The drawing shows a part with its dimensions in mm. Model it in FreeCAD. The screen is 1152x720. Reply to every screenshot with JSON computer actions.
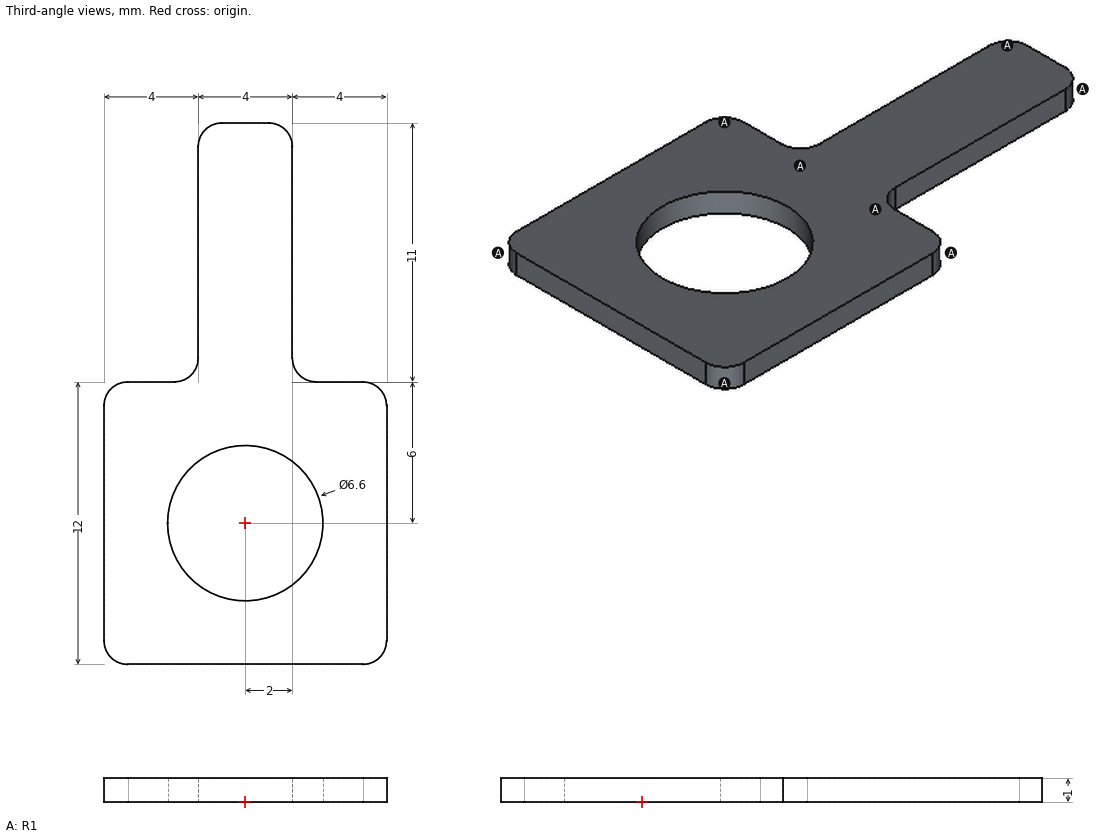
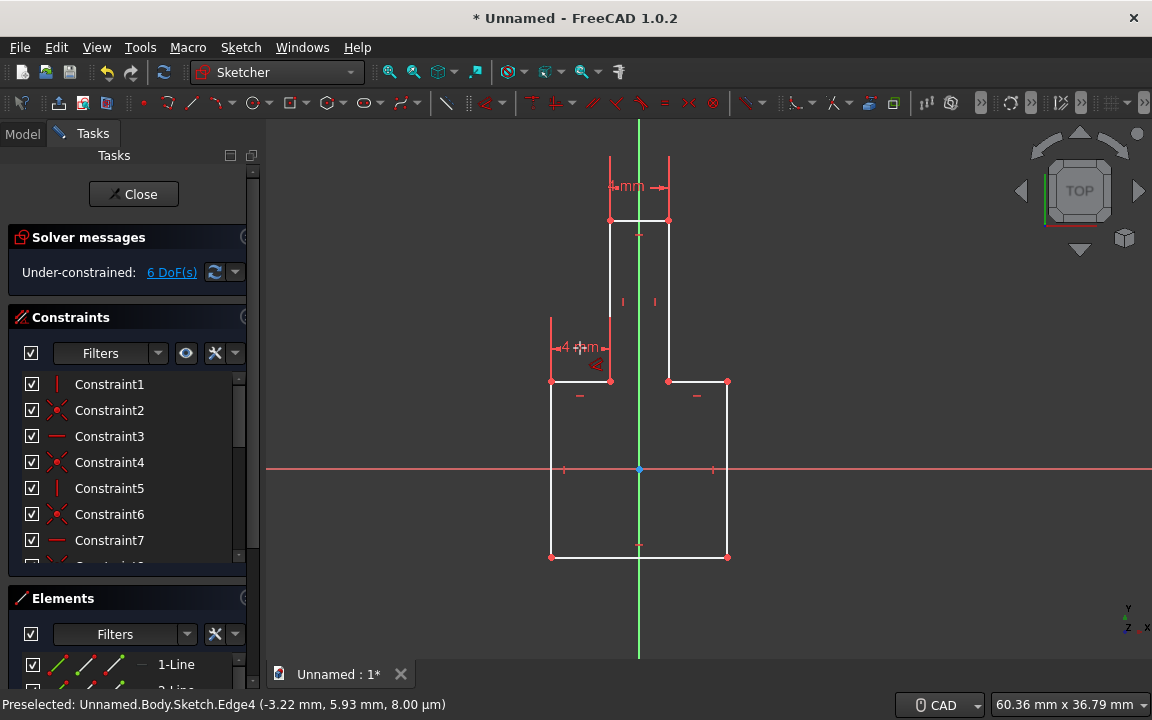
{"action": "left_click", "coordinate": [710, 382]}
{"action": "left_click", "coordinate": [698, 348]}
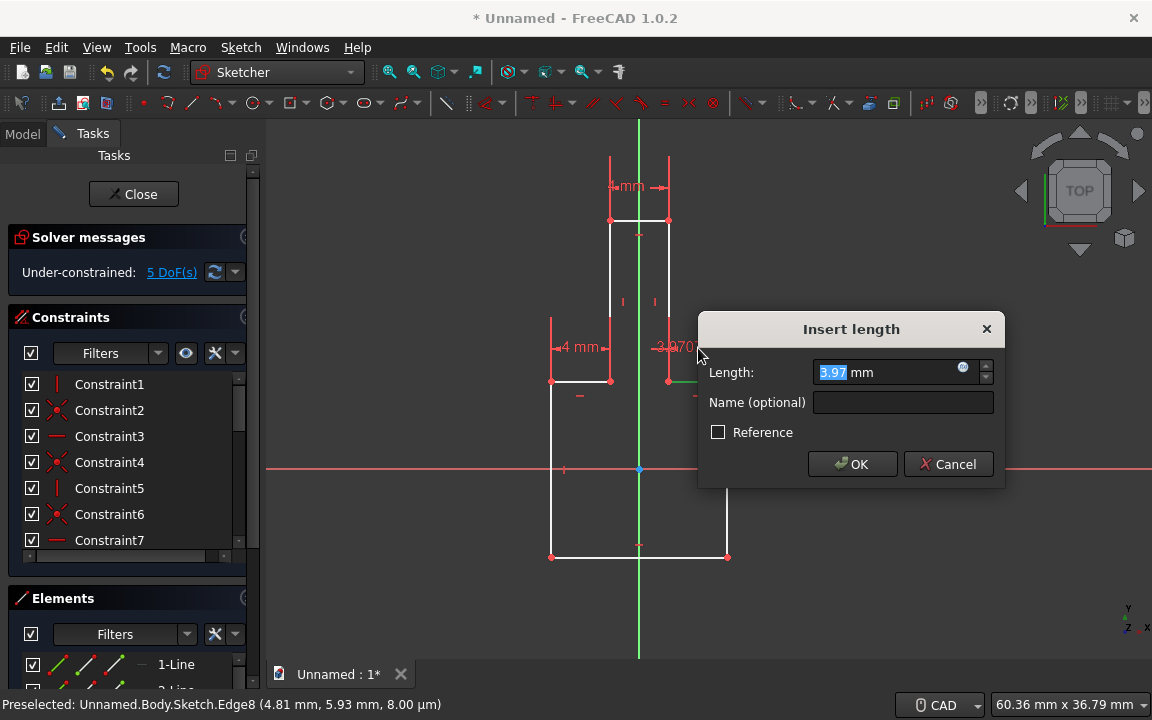
{"action": "type", "text": "4"}
{"action": "key", "text": "Return"}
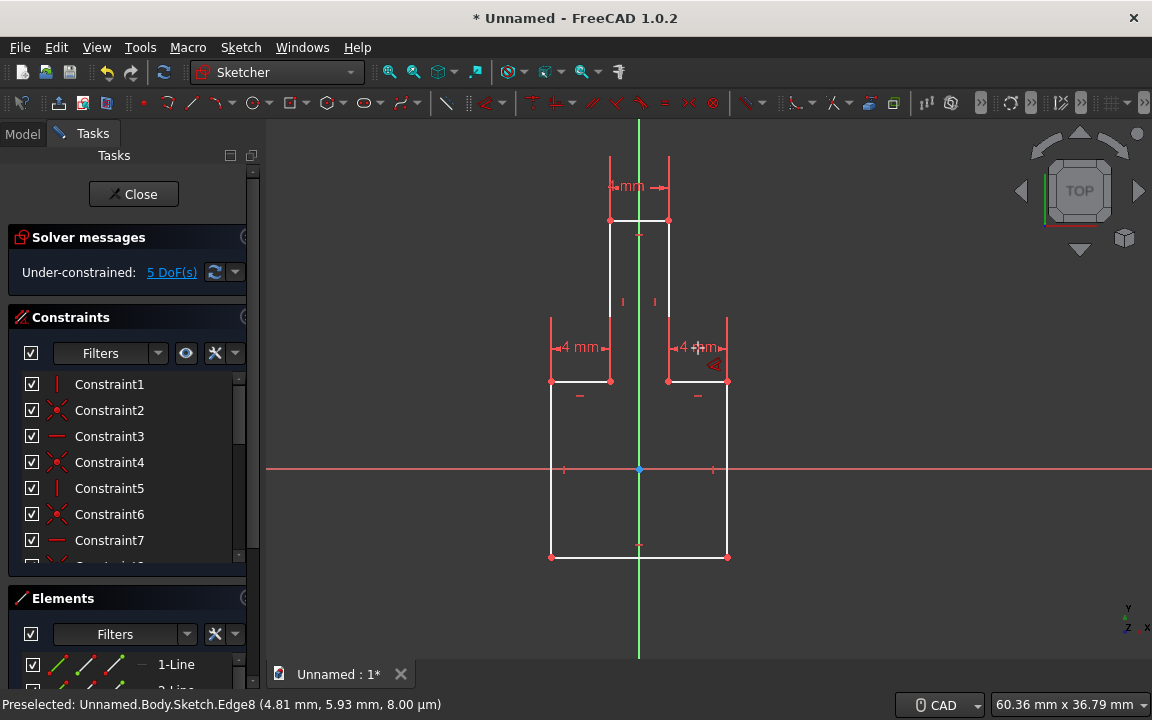
{"action": "left_click", "coordinate": [669, 334]}
{"action": "left_click", "coordinate": [703, 302]}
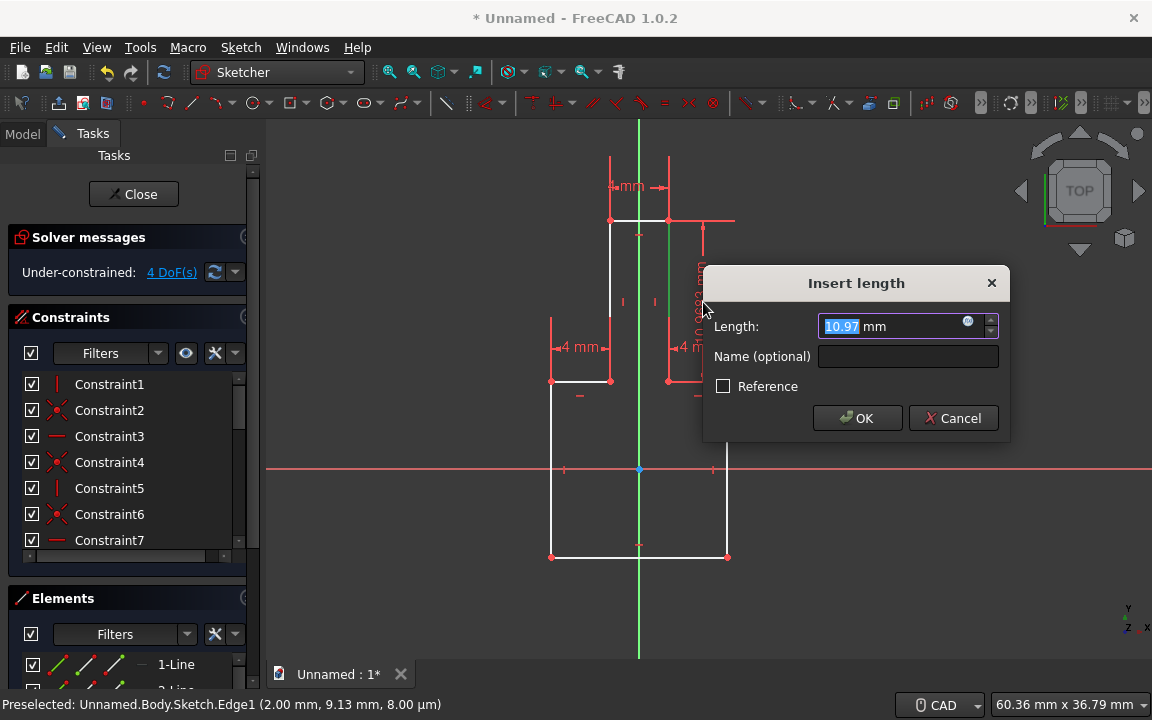
{"action": "type", "text": "11"}
{"action": "key", "text": "Return"}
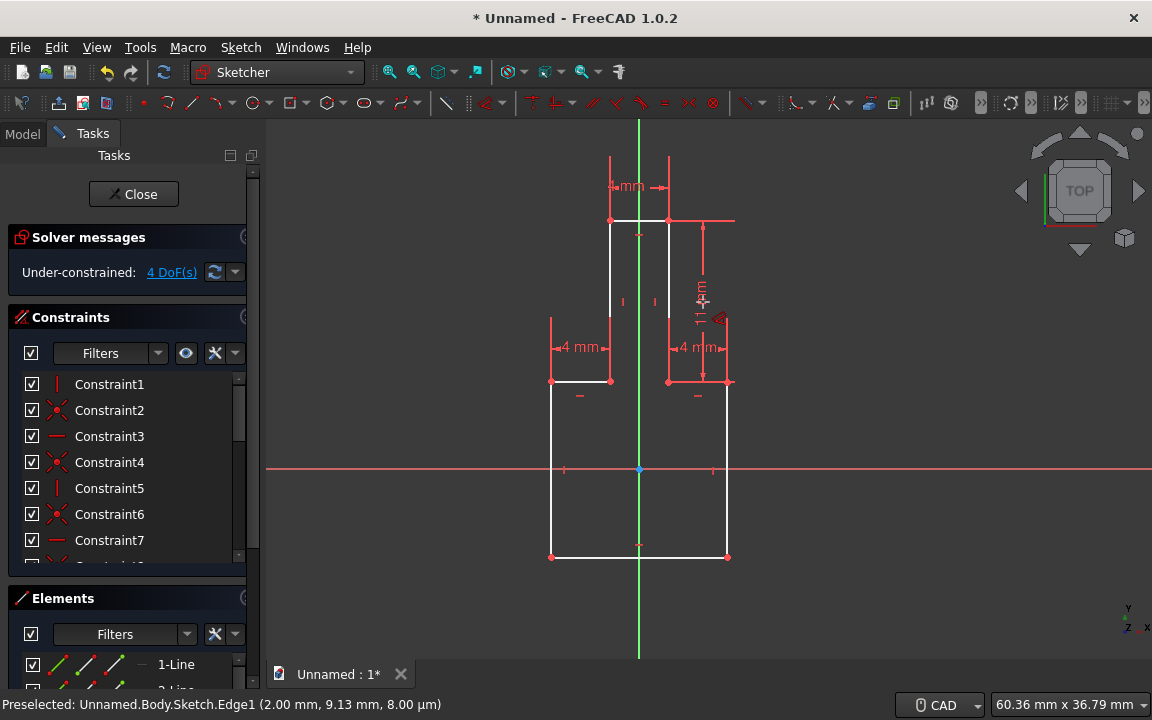
{"action": "left_click", "coordinate": [610, 269]}
{"action": "left_click", "coordinate": [576, 302]}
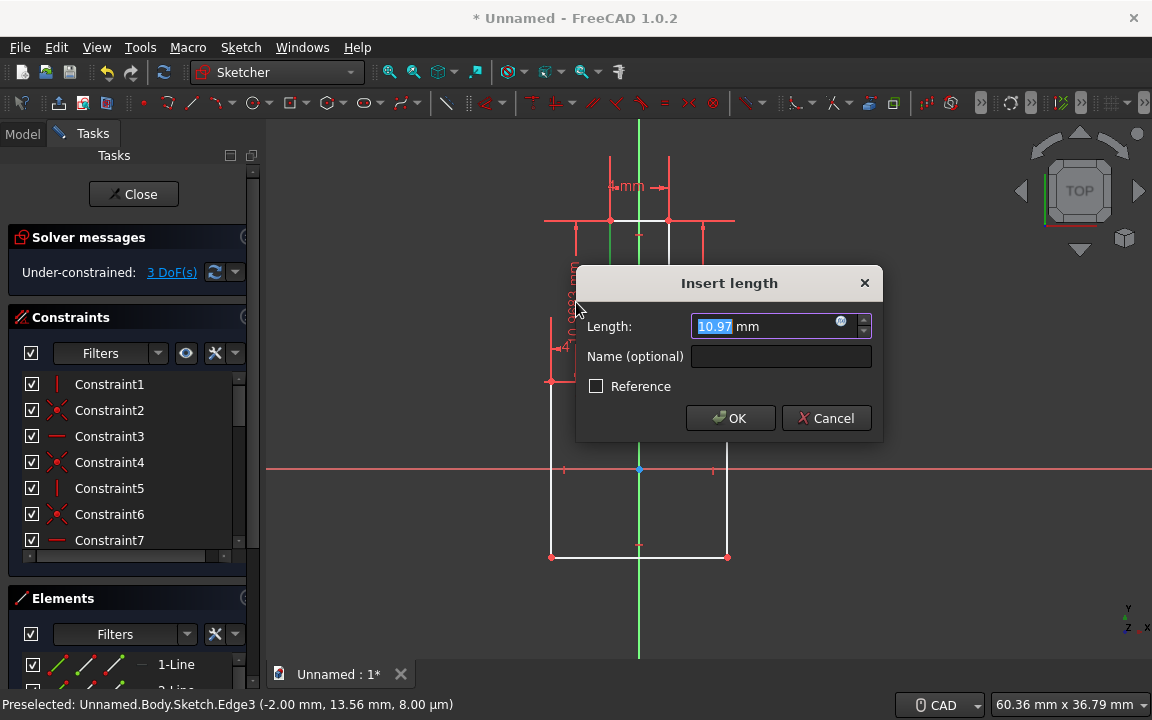
{"action": "type", "text": "11"}
{"action": "key", "text": "Return"}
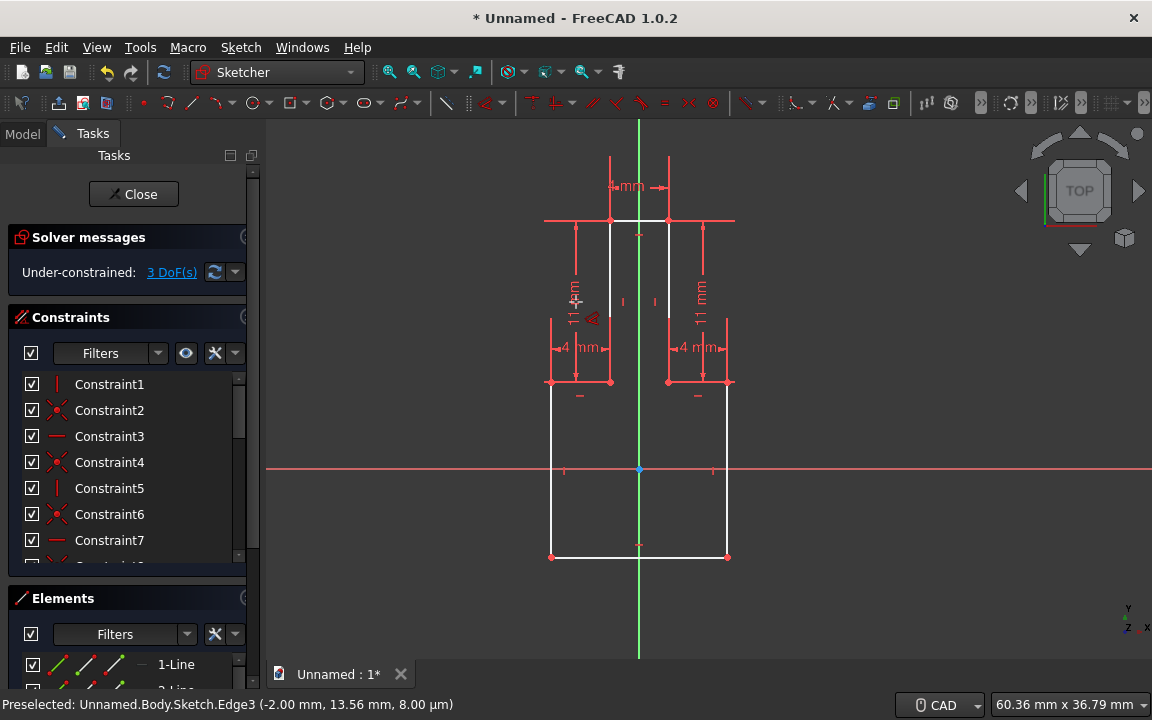
{"action": "left_click", "coordinate": [551, 435]}
{"action": "left_click", "coordinate": [517, 430]}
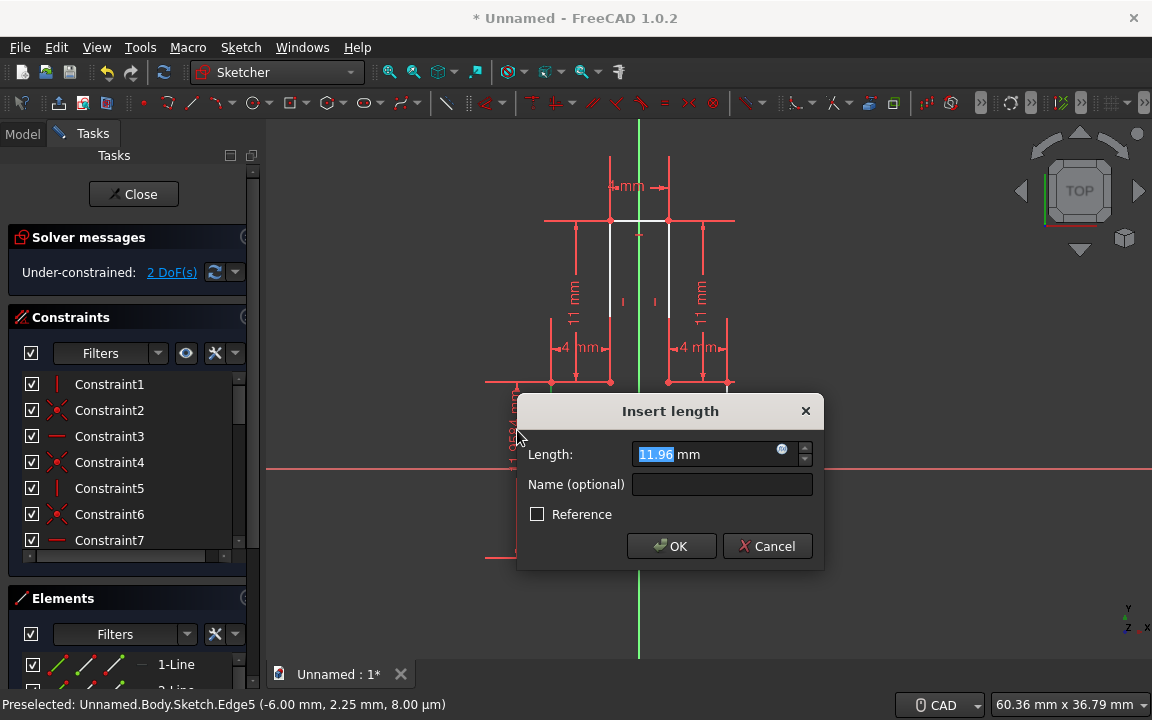
{"action": "type", "text": "12"}
{"action": "key", "text": "Return"}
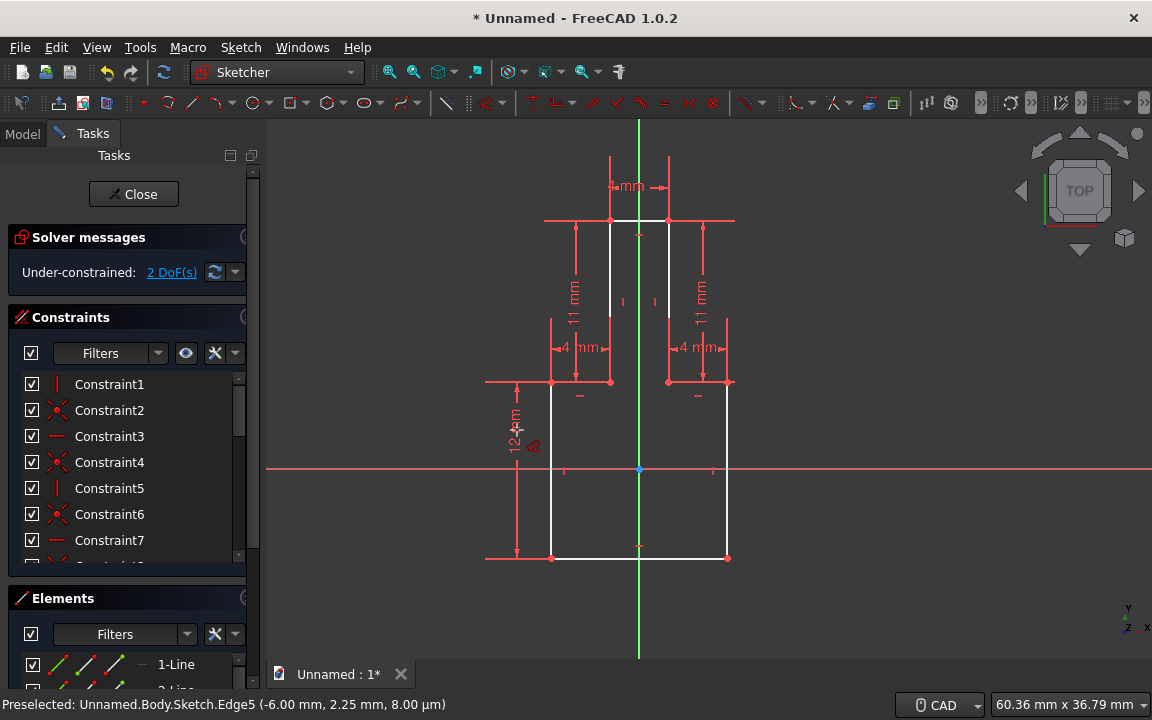
{"action": "scroll", "coordinate": [669, 382], "scroll_direction": "up", "scroll_amount": 2}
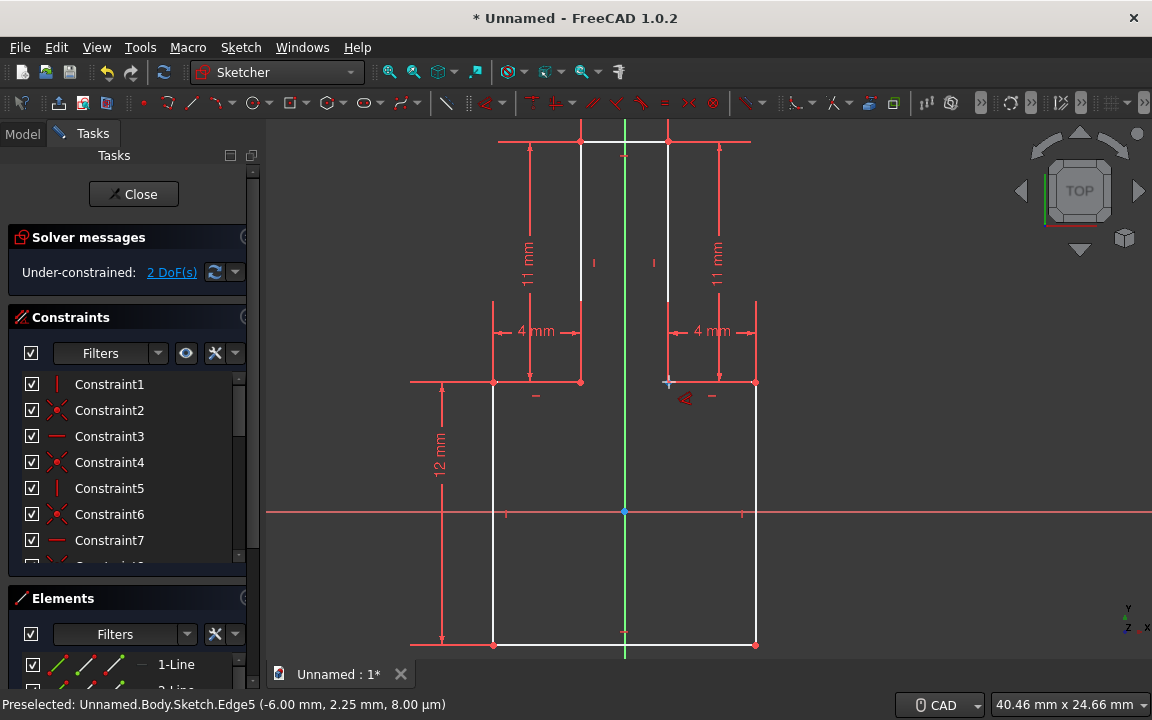
{"action": "left_click", "coordinate": [668, 382]}
{"action": "left_click", "coordinate": [646, 546]}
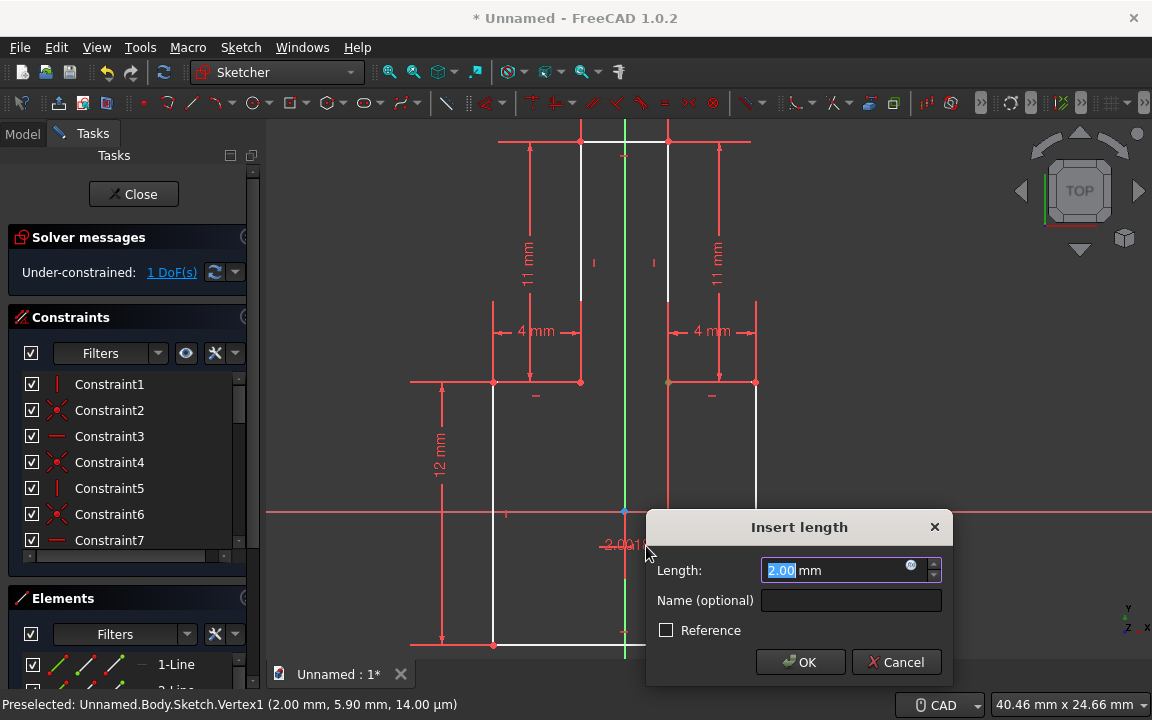
{"action": "type", "text": "2"}
{"action": "key", "text": "Return"}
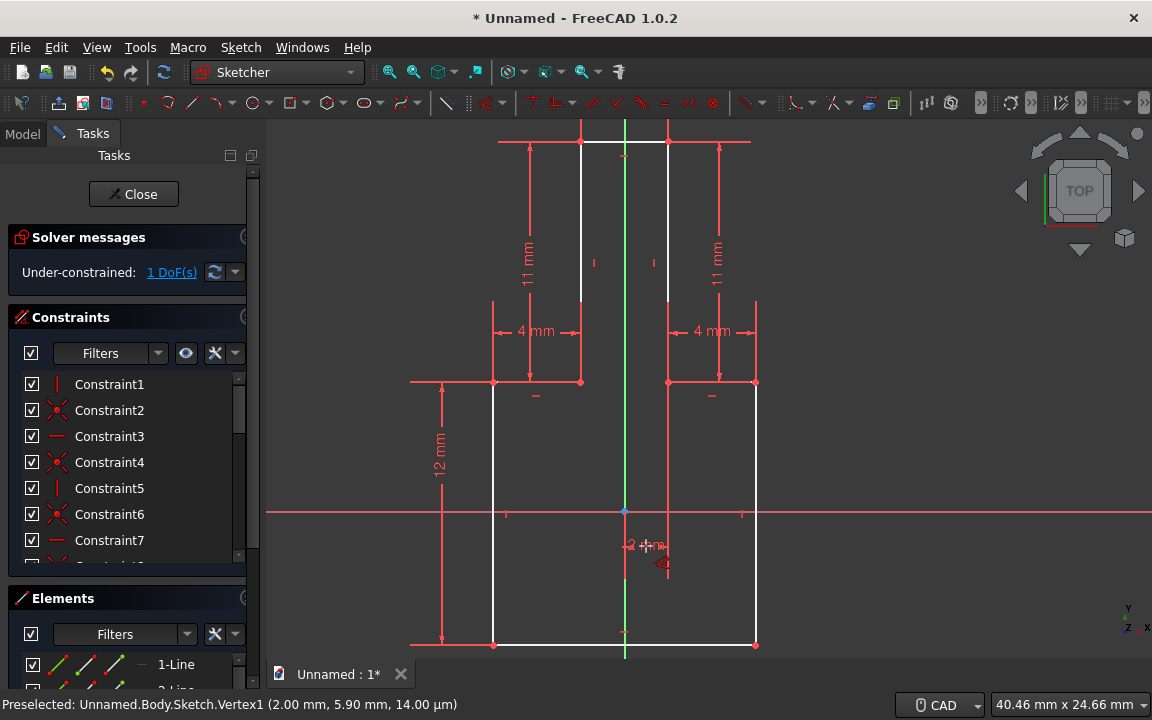
{"action": "left_click", "coordinate": [668, 382]}
{"action": "left_click", "coordinate": [702, 447]}